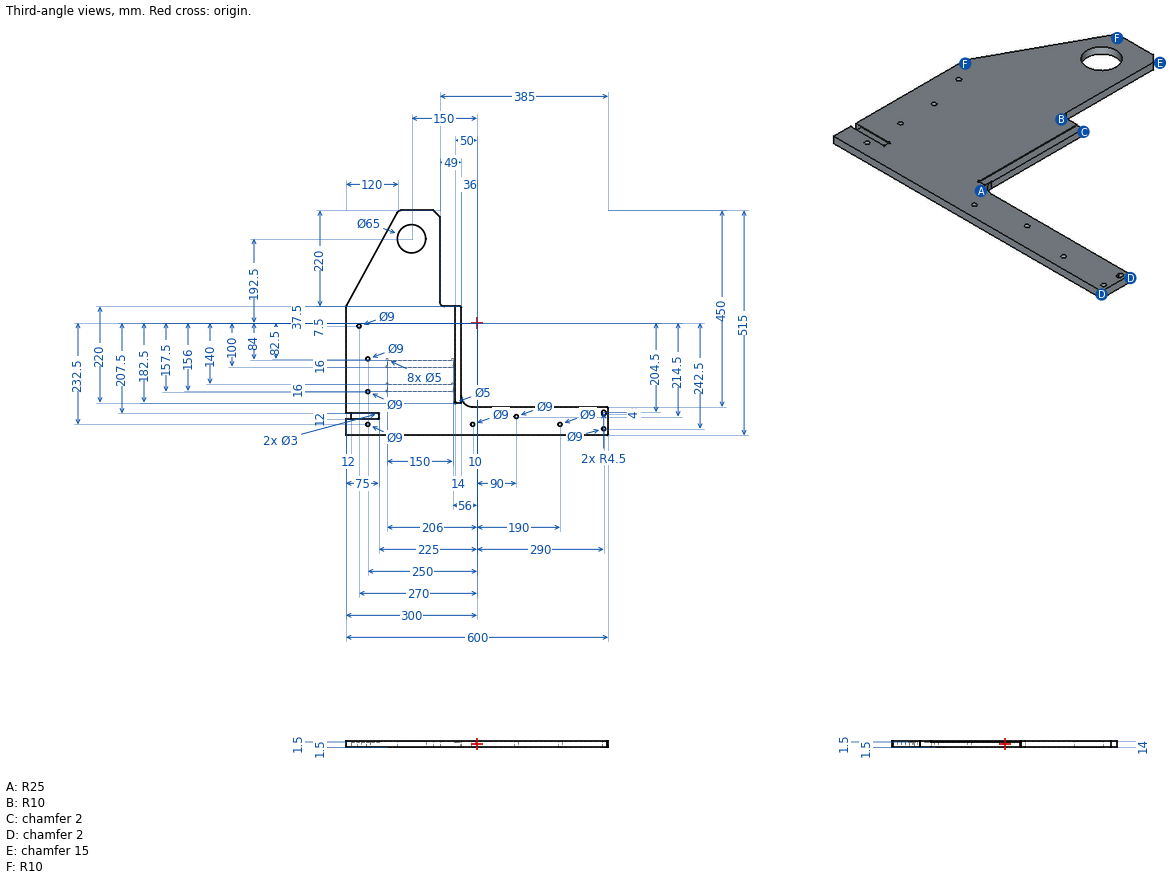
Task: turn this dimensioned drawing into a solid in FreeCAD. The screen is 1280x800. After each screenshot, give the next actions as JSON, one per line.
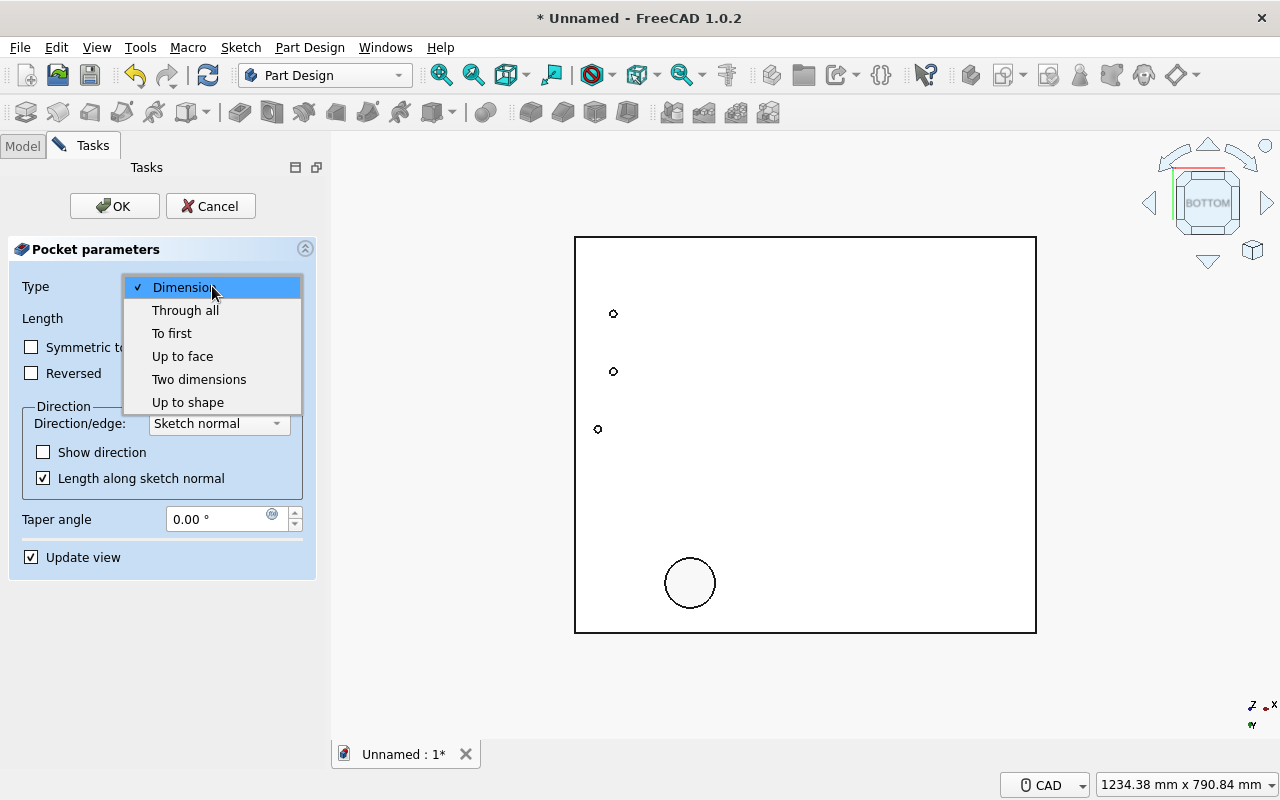
{"action": "left_click", "coordinate": [212, 334]}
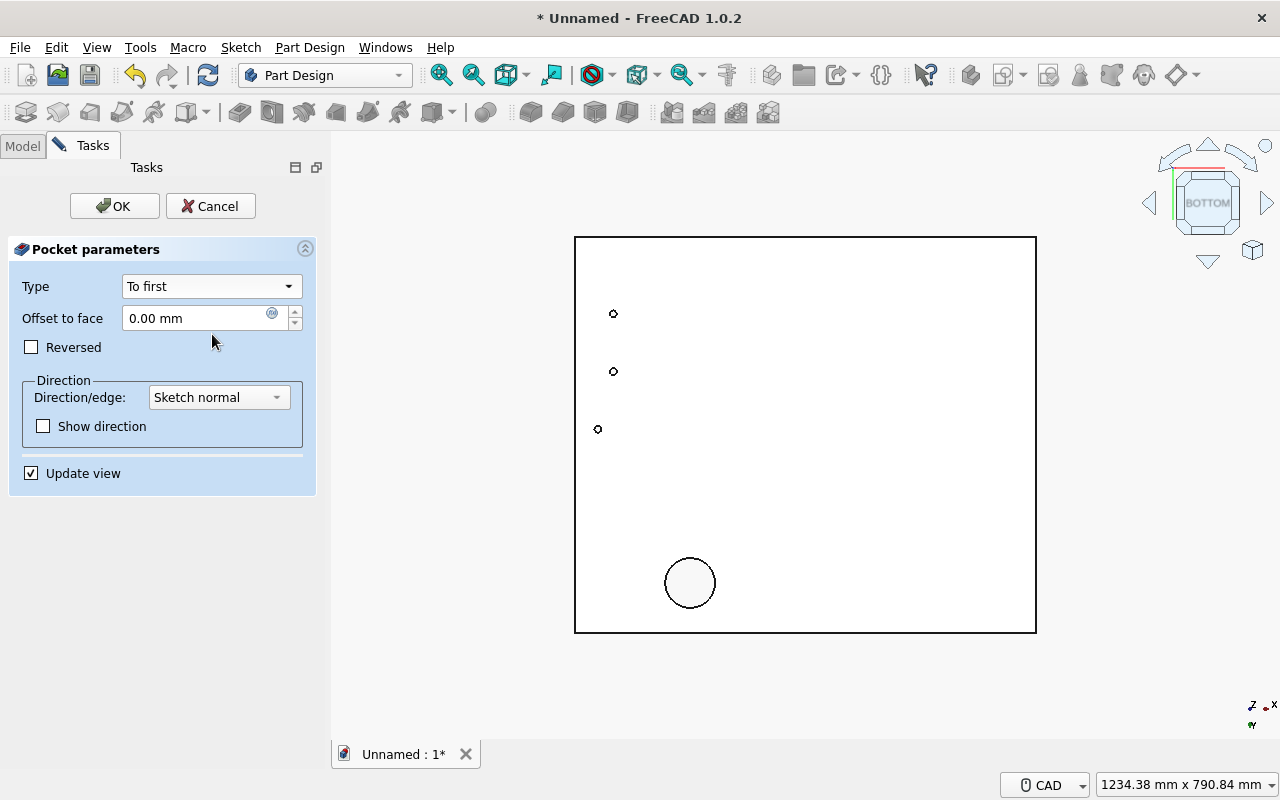
{"action": "left_click", "coordinate": [115, 206]}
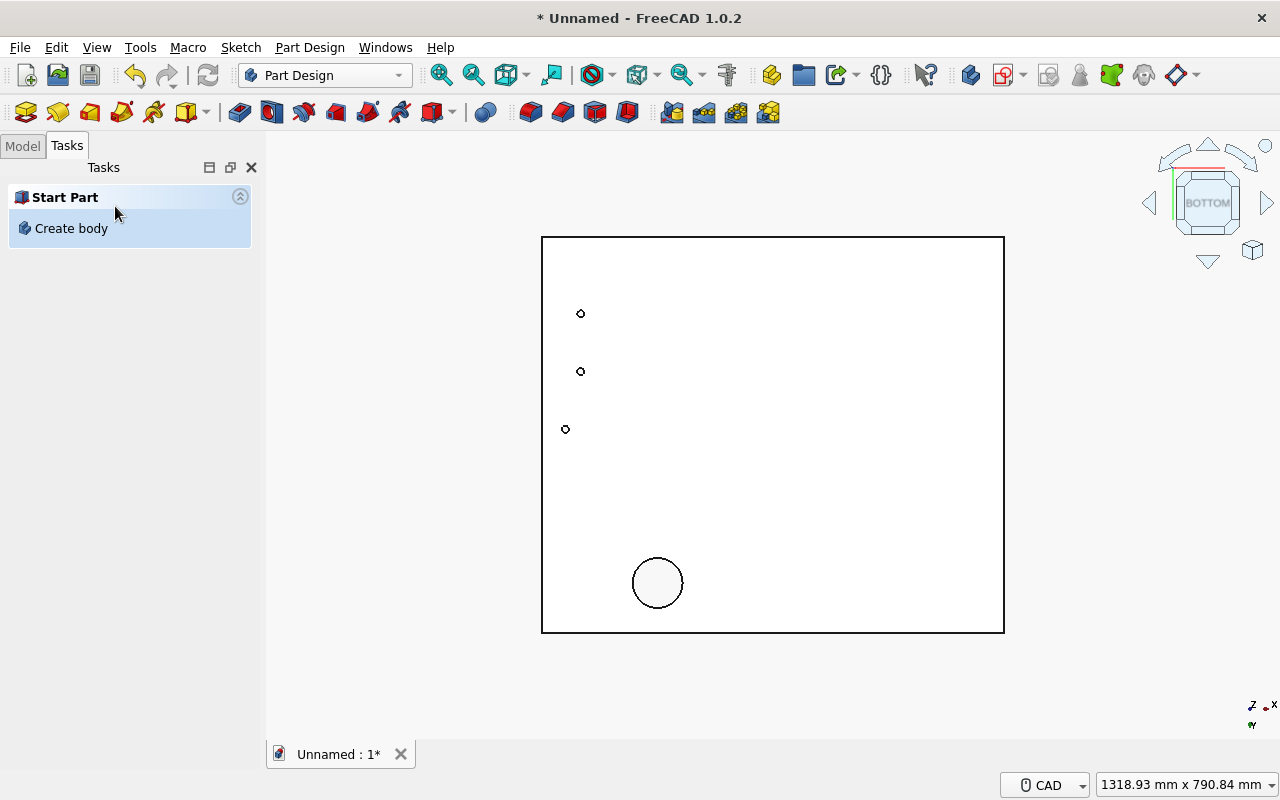
{"action": "left_click", "coordinate": [839, 434]}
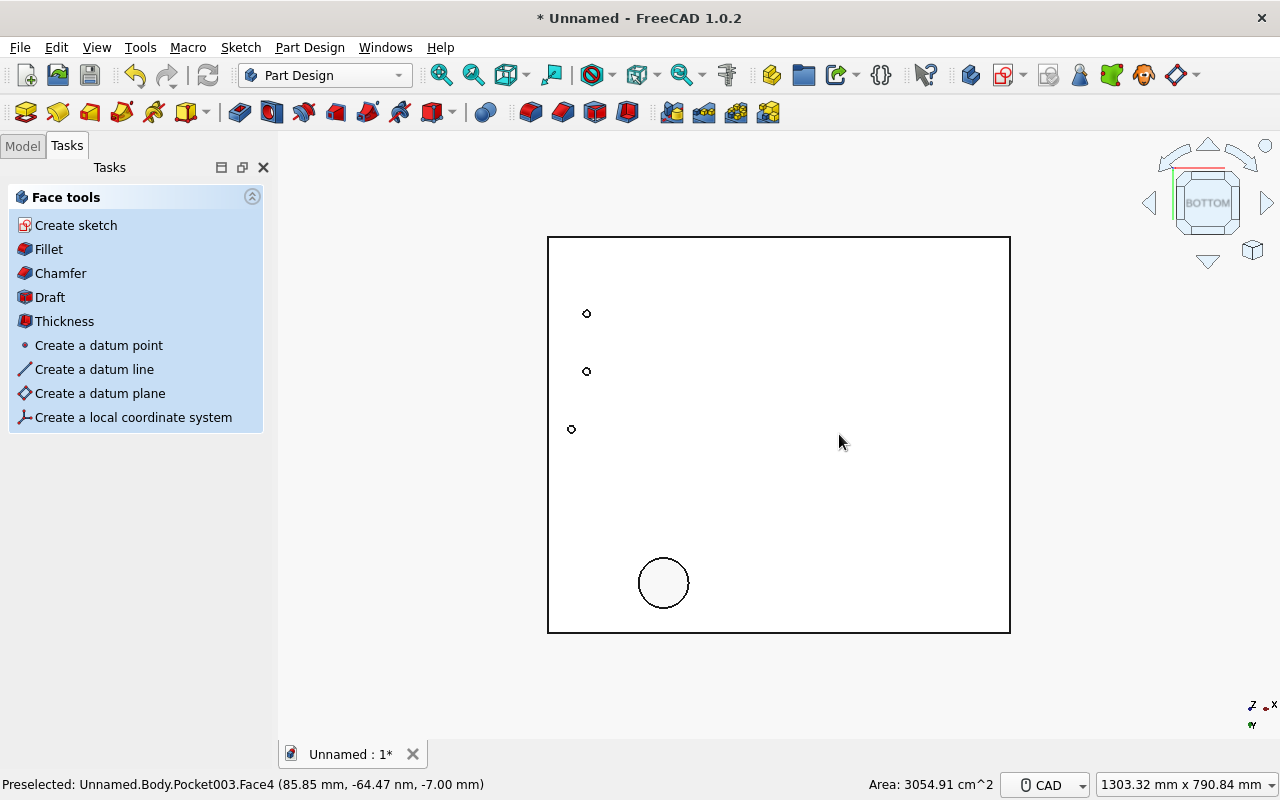
{"action": "left_click", "coordinate": [1004, 76]}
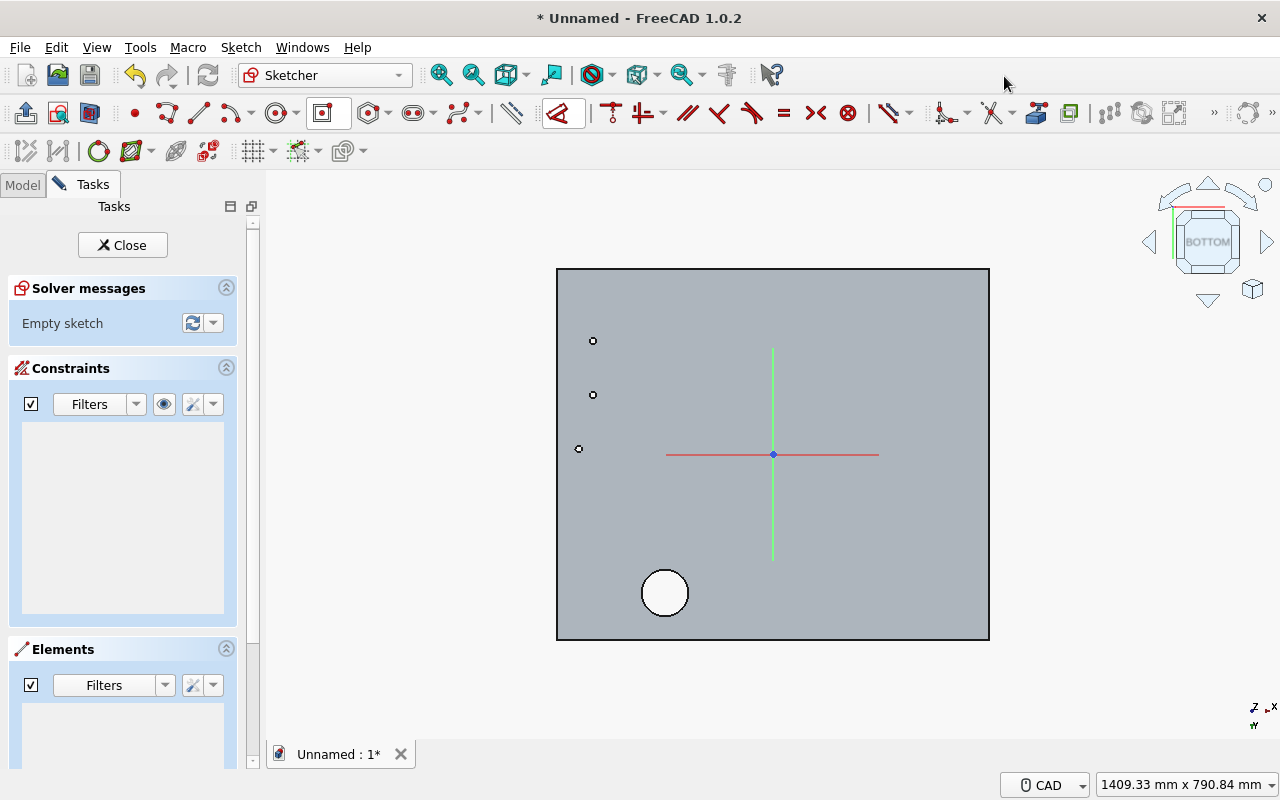
{"action": "scroll", "coordinate": [587, 278], "scroll_direction": "up", "scroll_amount": 15}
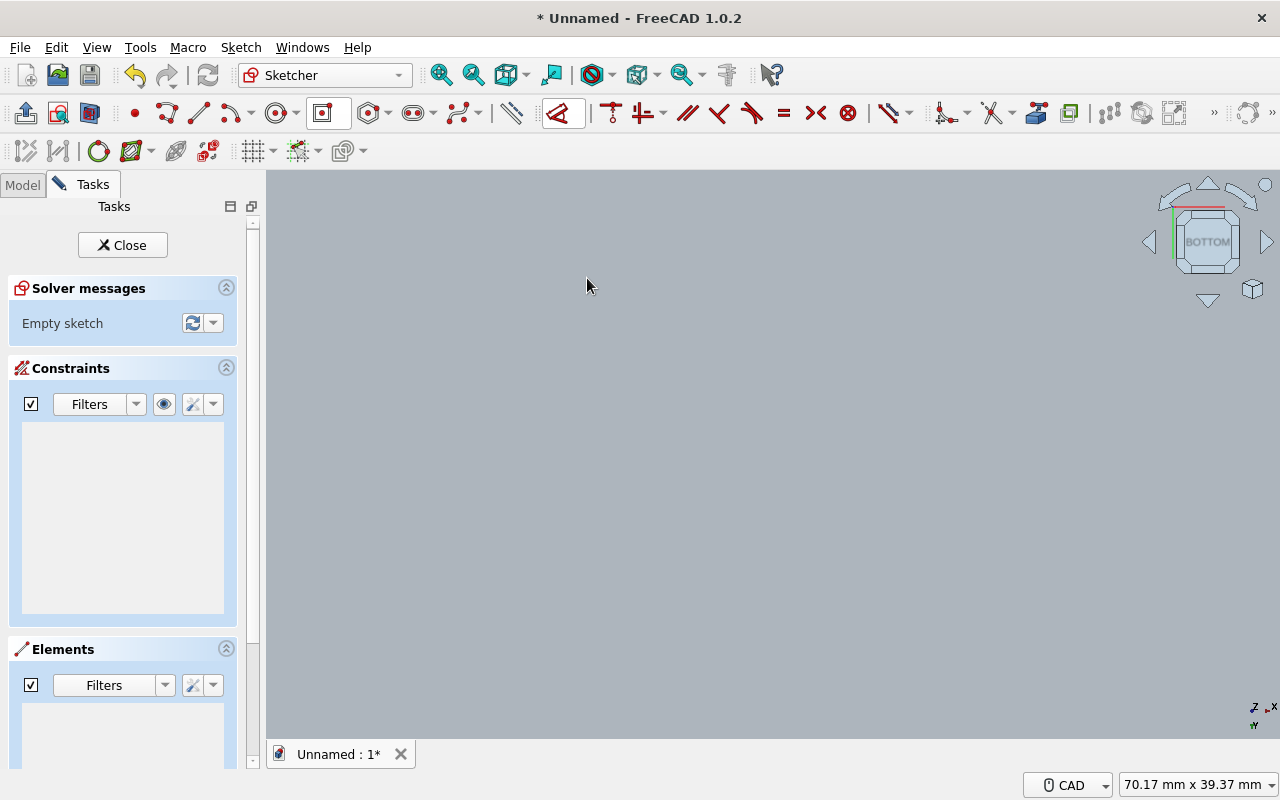
{"action": "scroll", "coordinate": [704, 462], "scroll_direction": "up", "scroll_amount": 5}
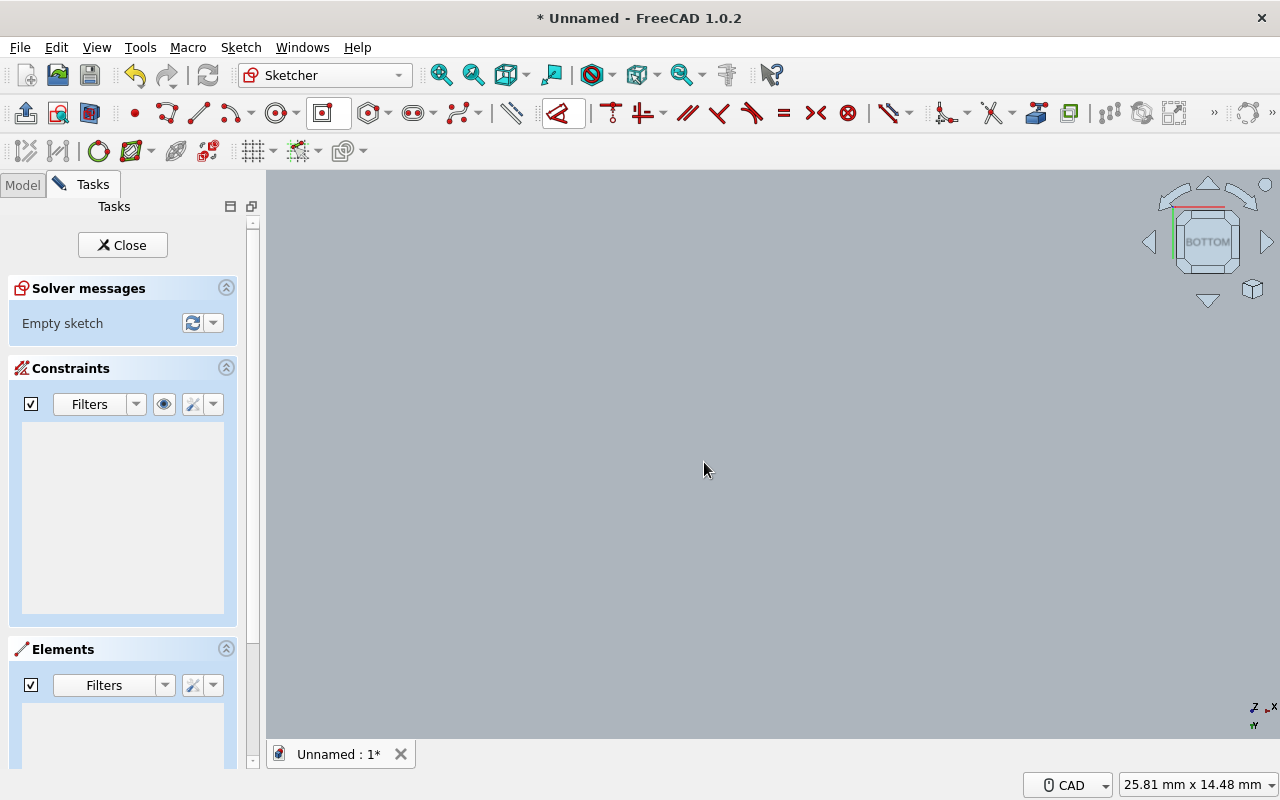
{"action": "left_click", "coordinate": [276, 114]}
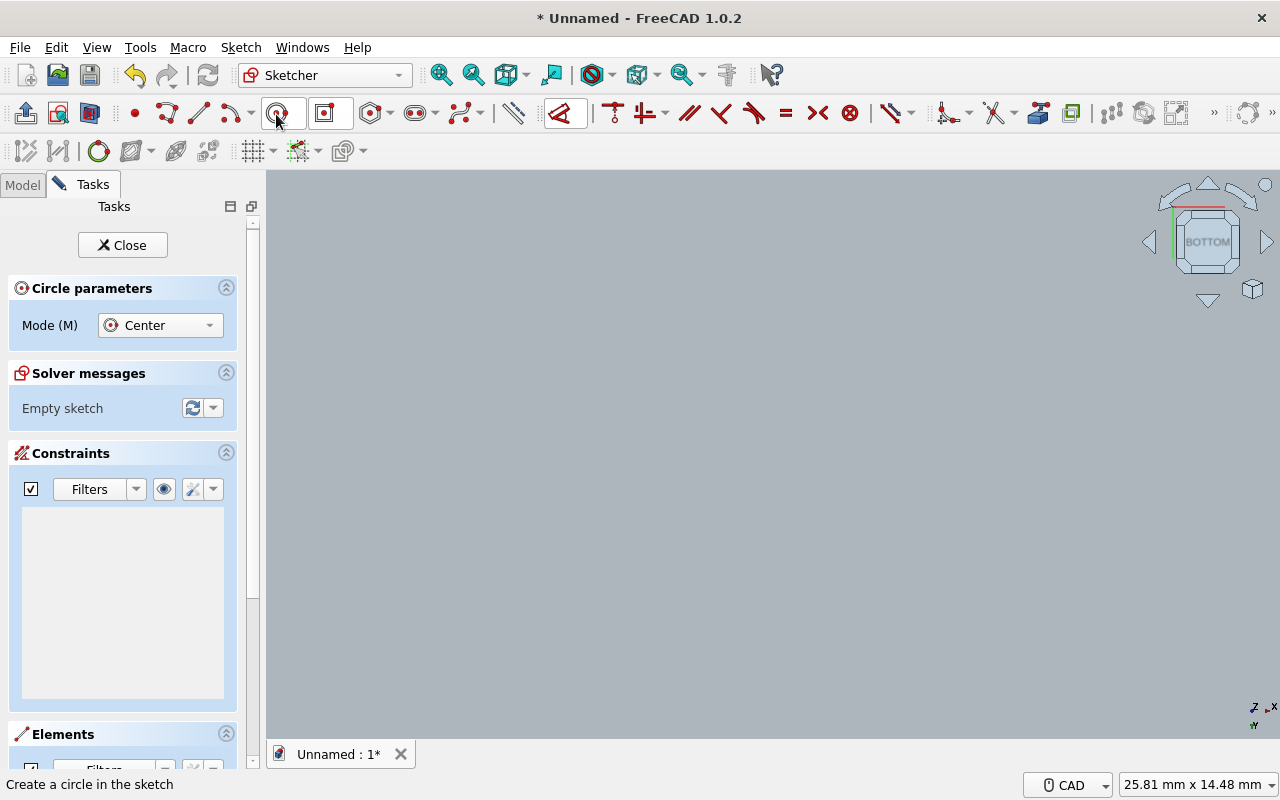
{"action": "left_click", "coordinate": [703, 454]}
{"action": "mouse_move", "coordinate": [828, 329]}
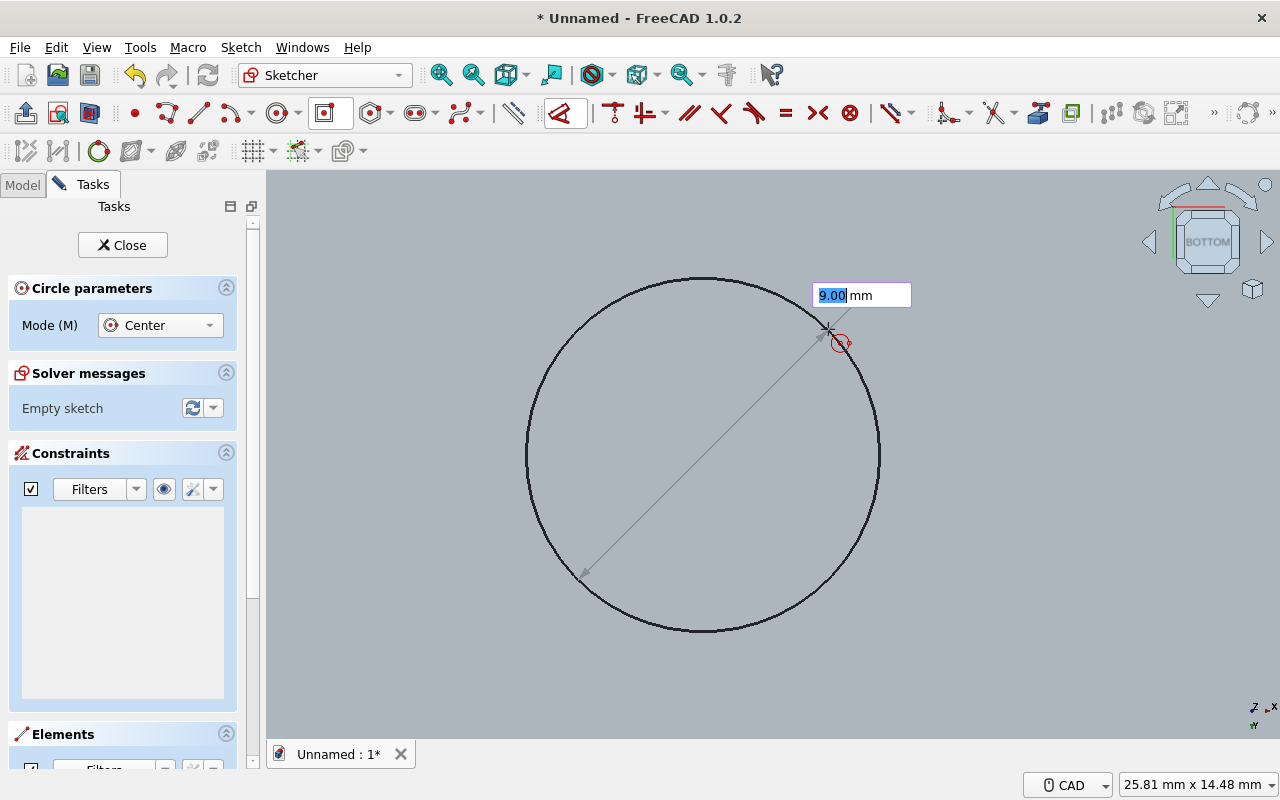
{"action": "type", "text": "9"}
{"action": "key", "text": "Return"}
{"action": "key", "text": "Escape"}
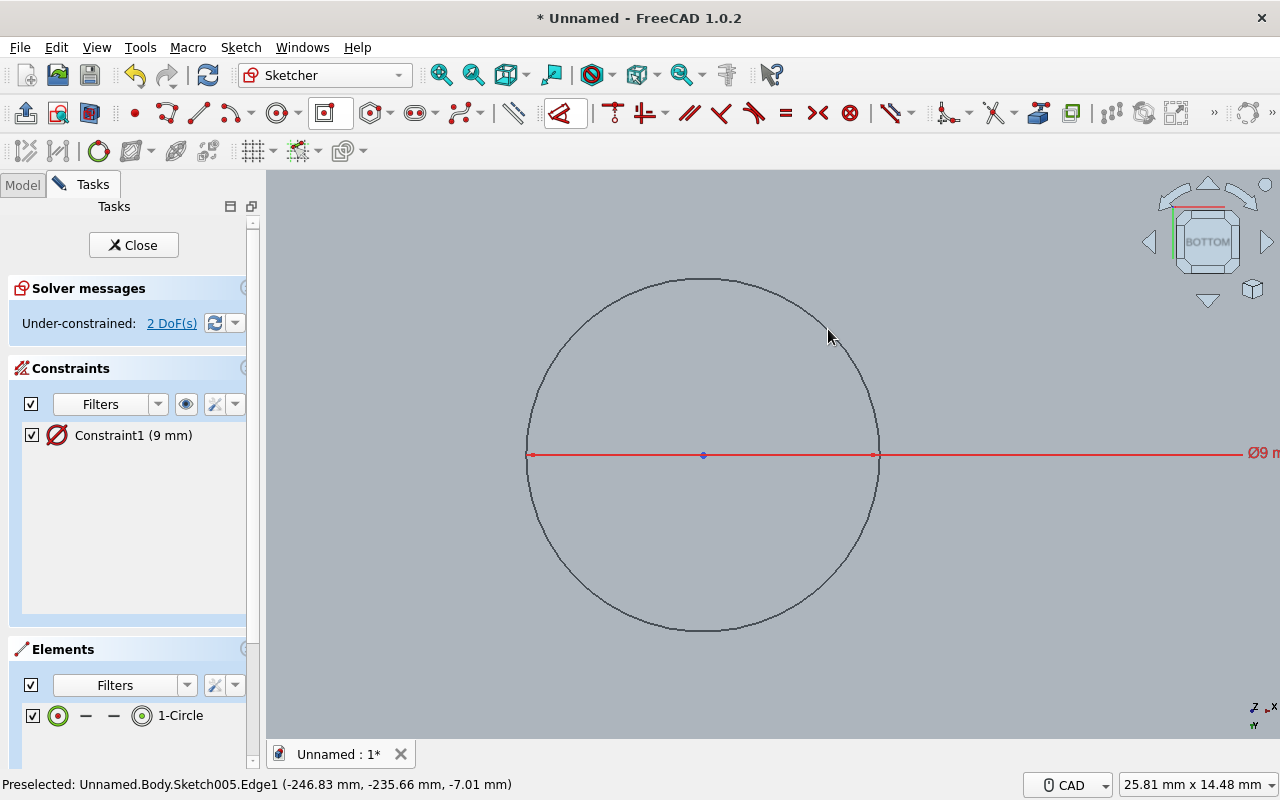
{"action": "left_click", "coordinate": [703, 455]}